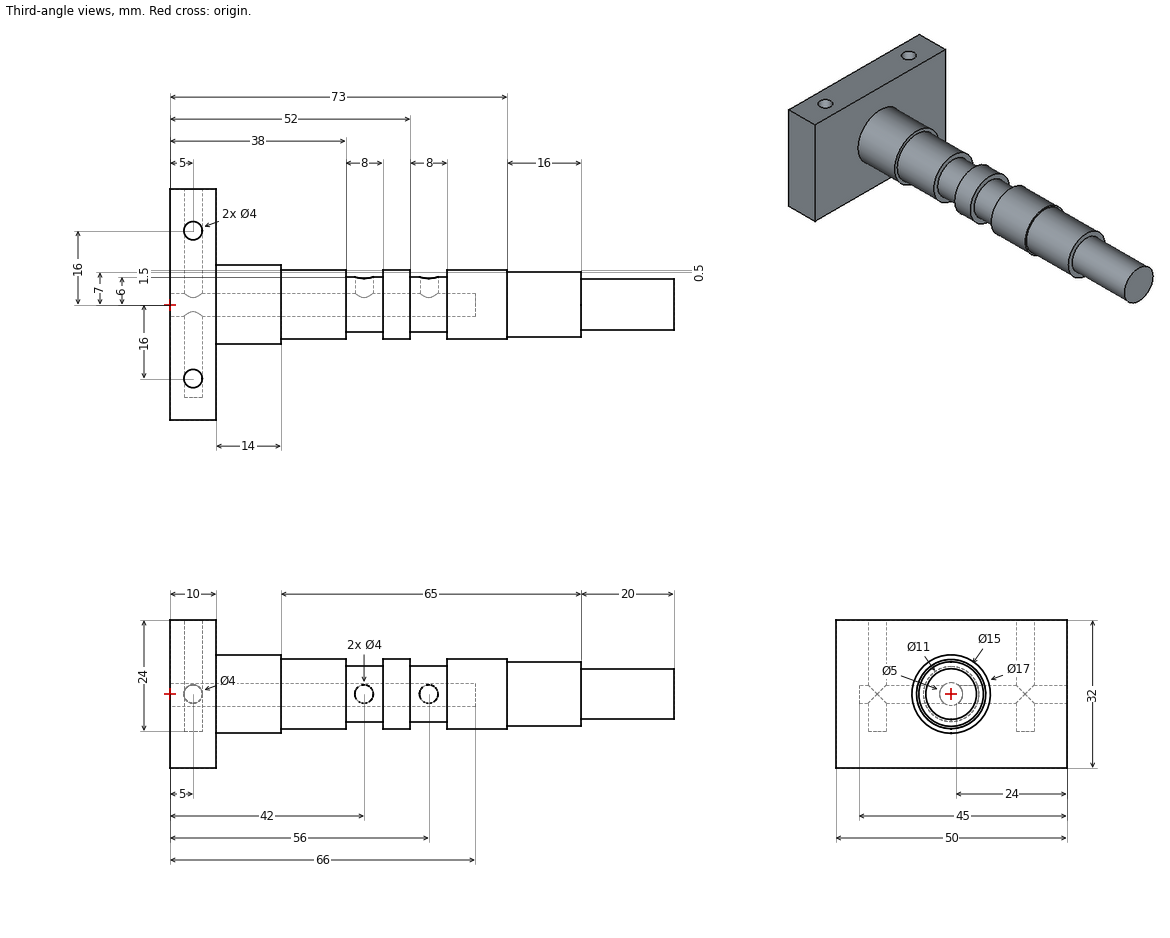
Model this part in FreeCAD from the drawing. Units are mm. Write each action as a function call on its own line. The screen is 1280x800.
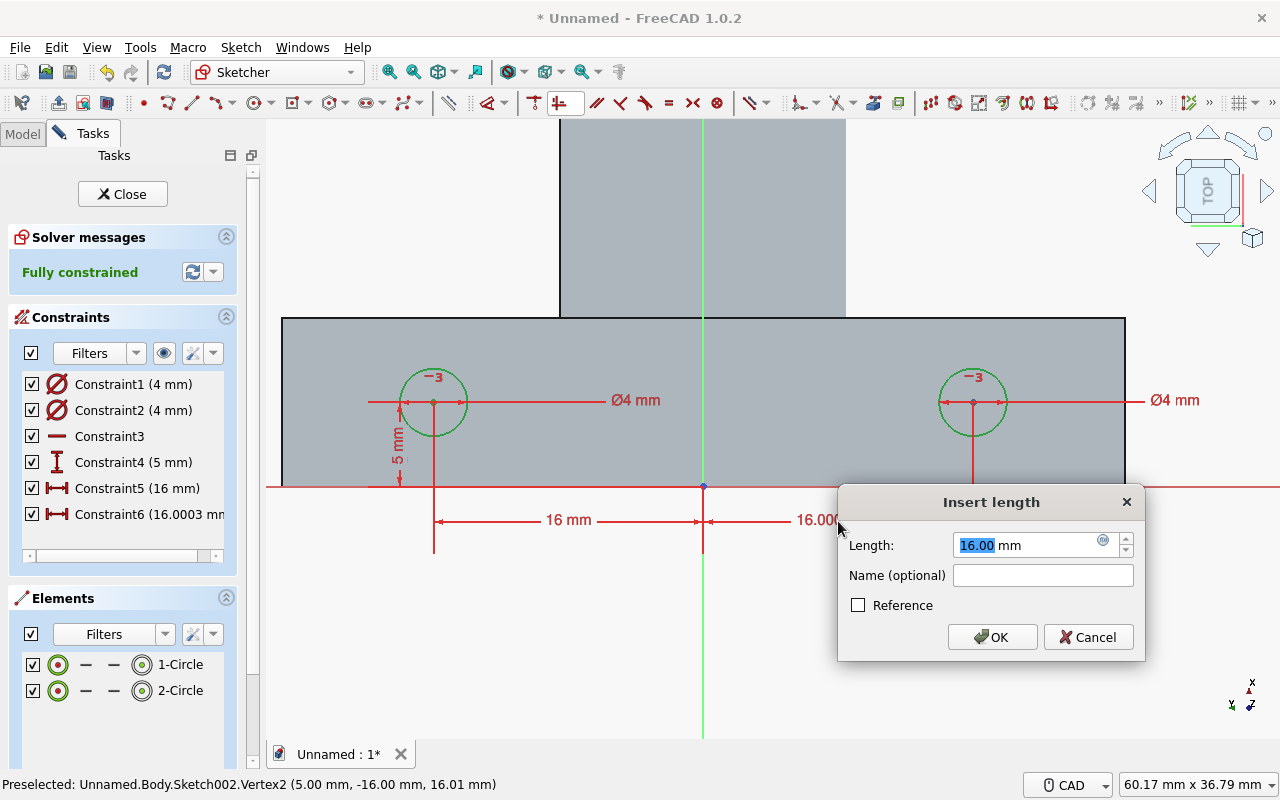
text(16)
key(Return)
key(Escape)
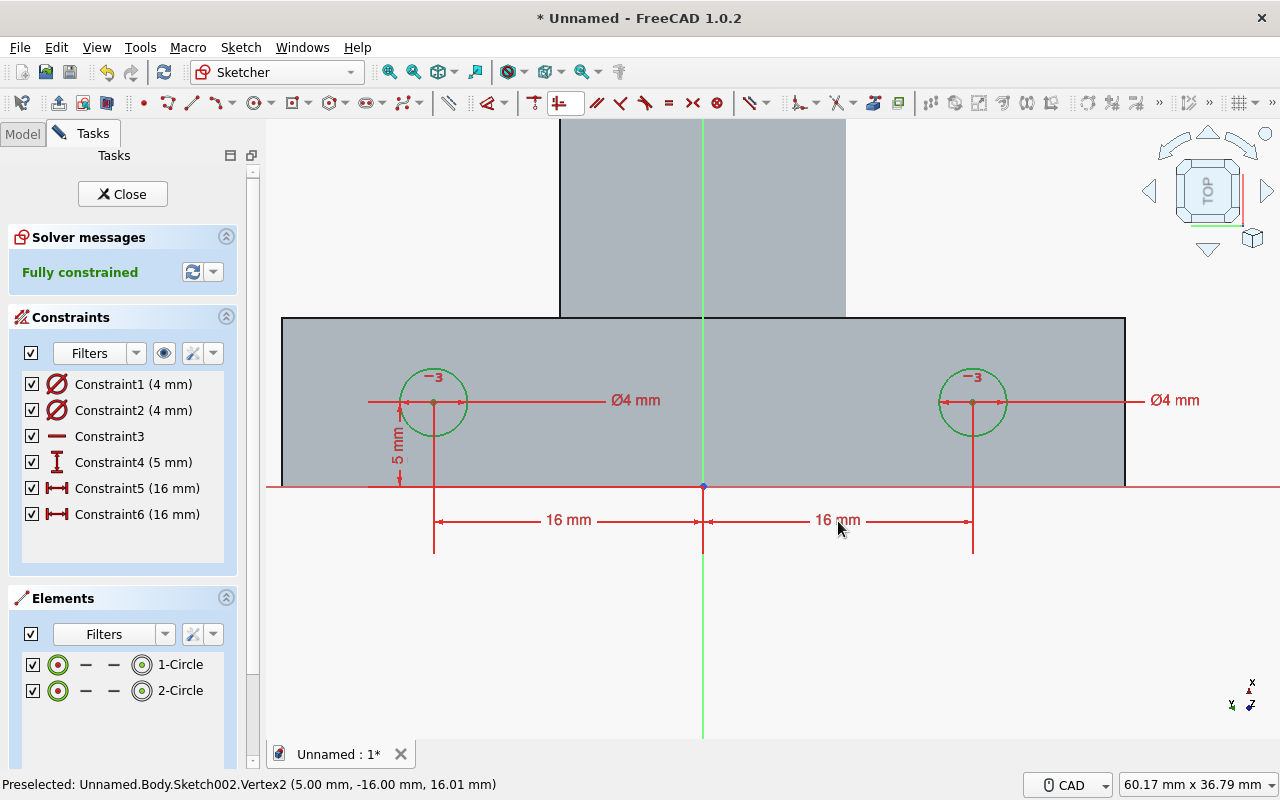
click(123, 194)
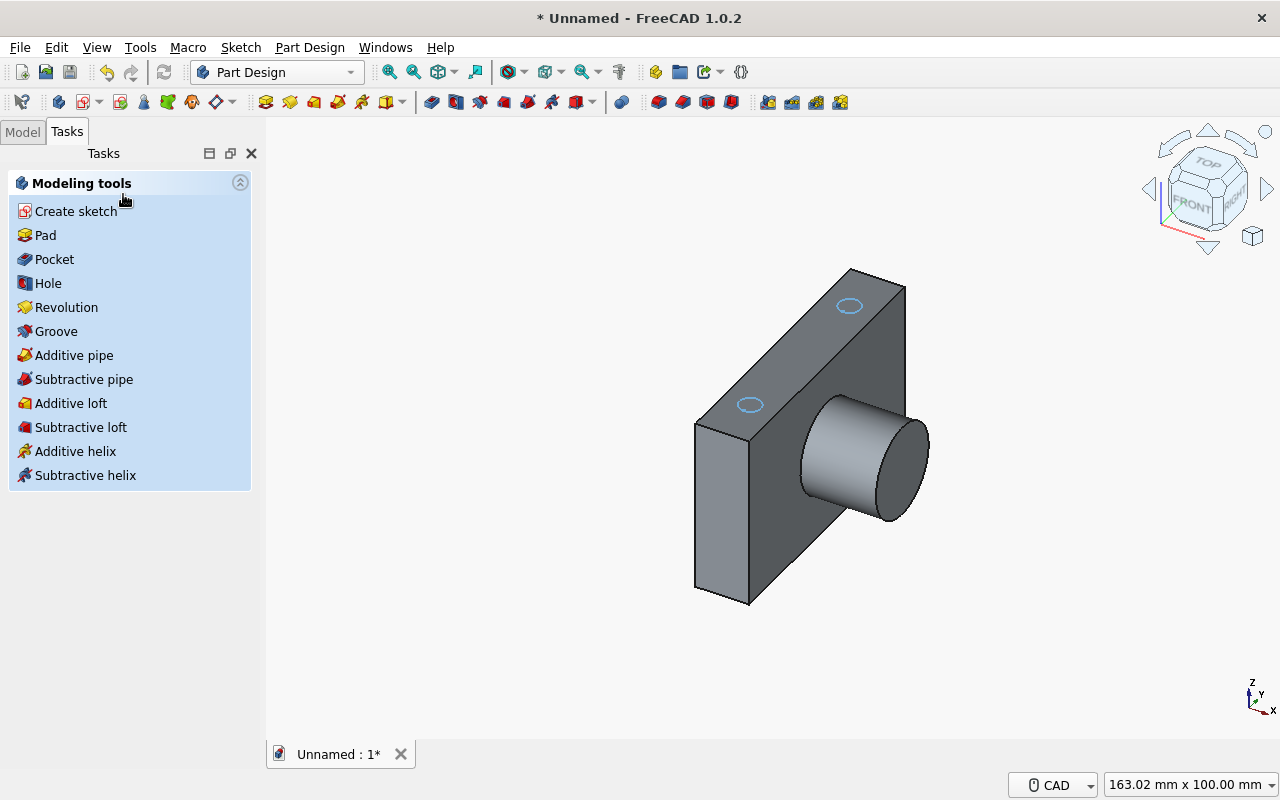
click(432, 102)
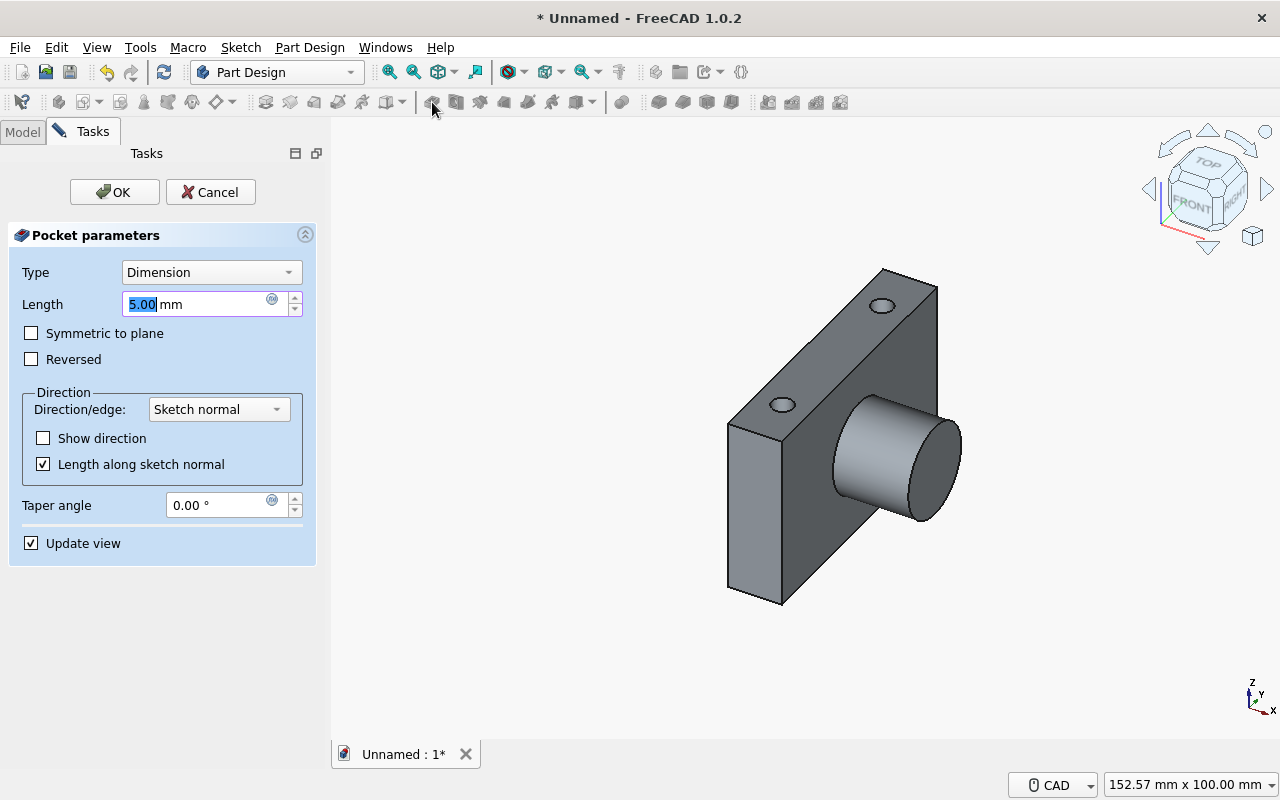
text(24)
key(Tab)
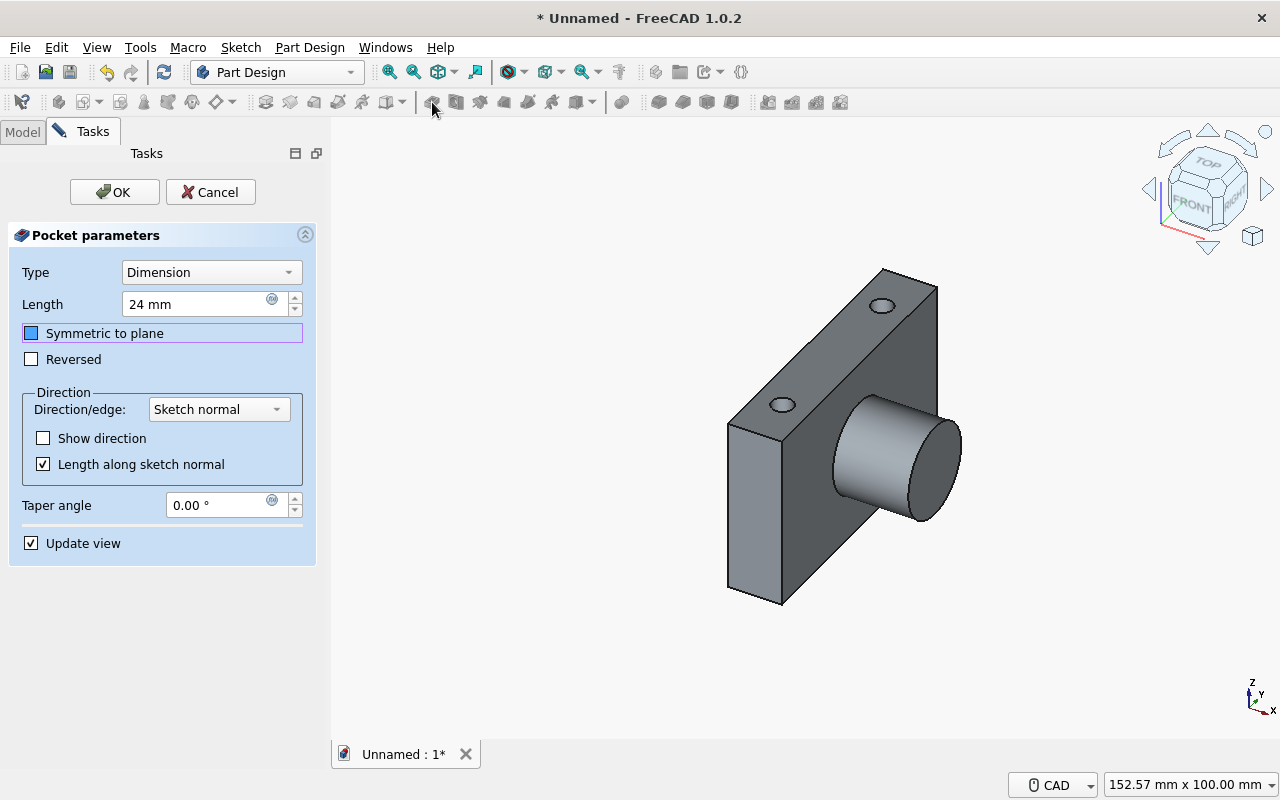
click(115, 192)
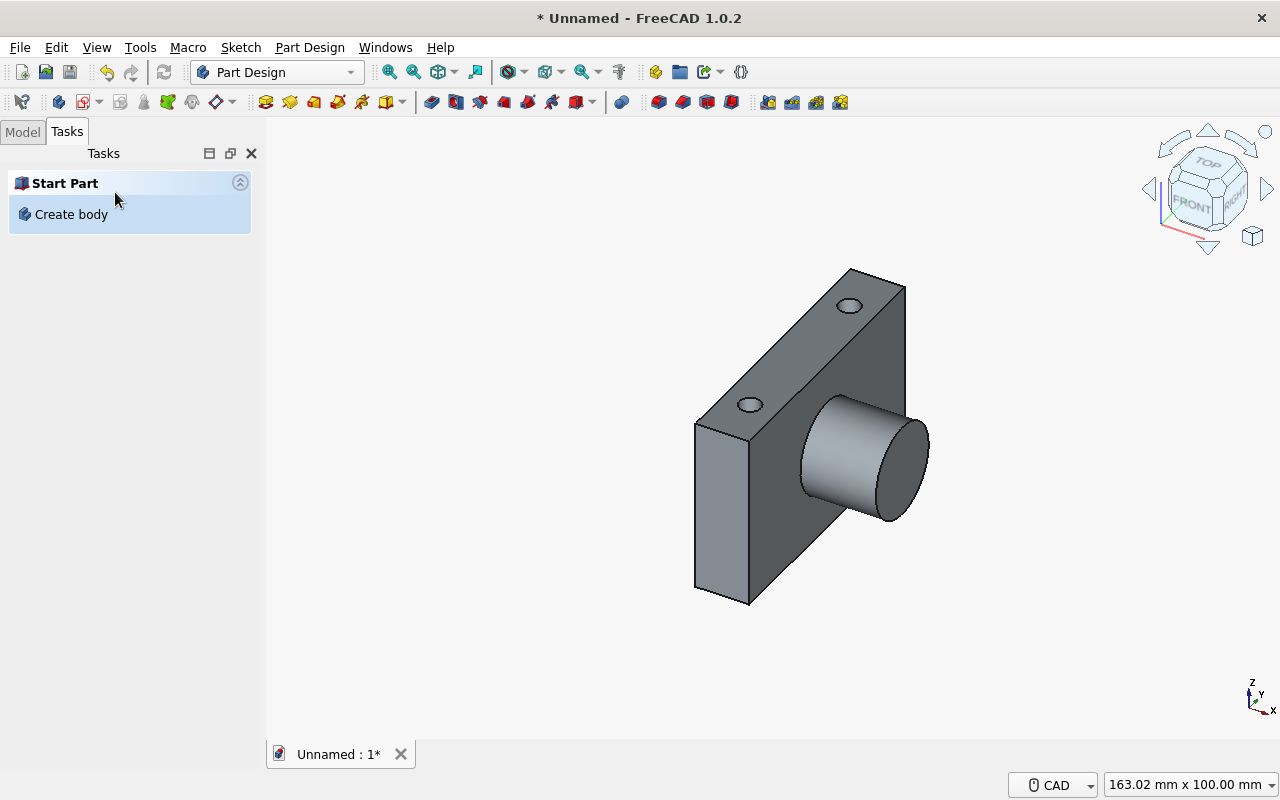
key(4)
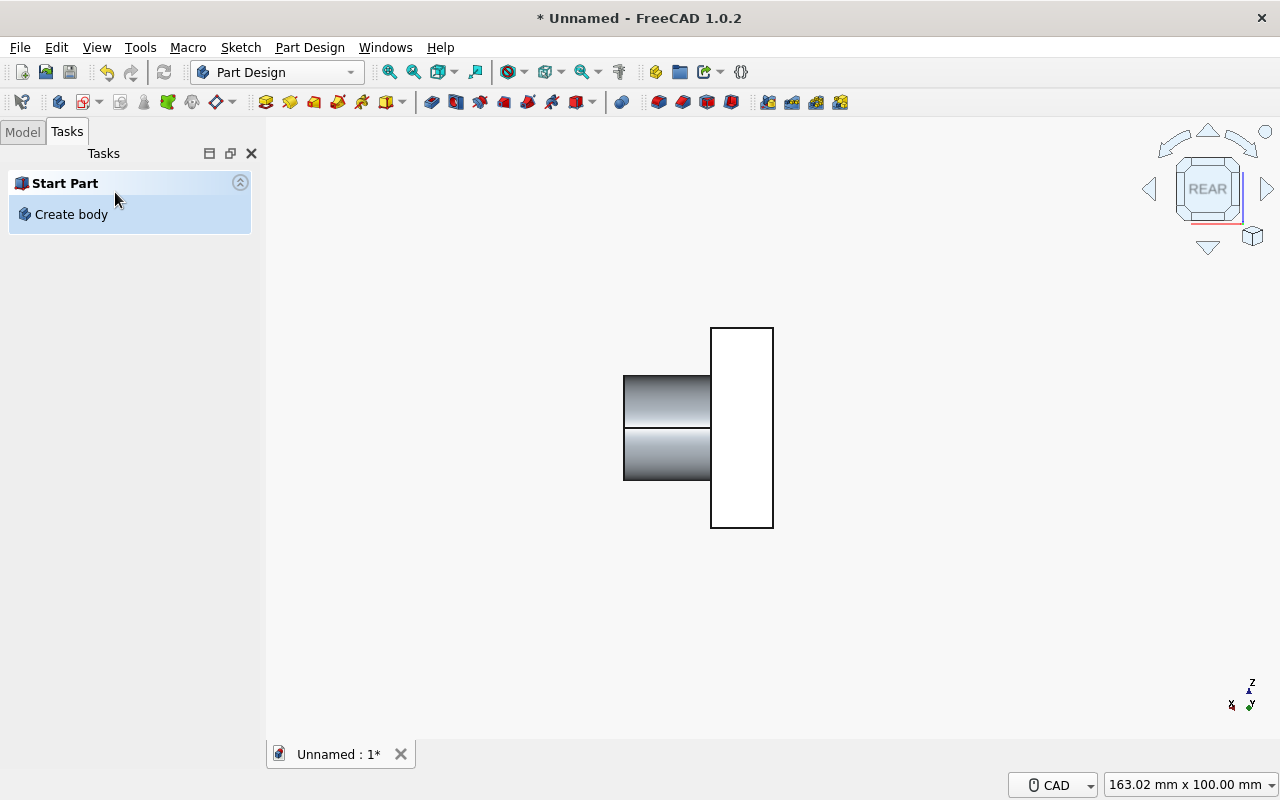
click(390, 72)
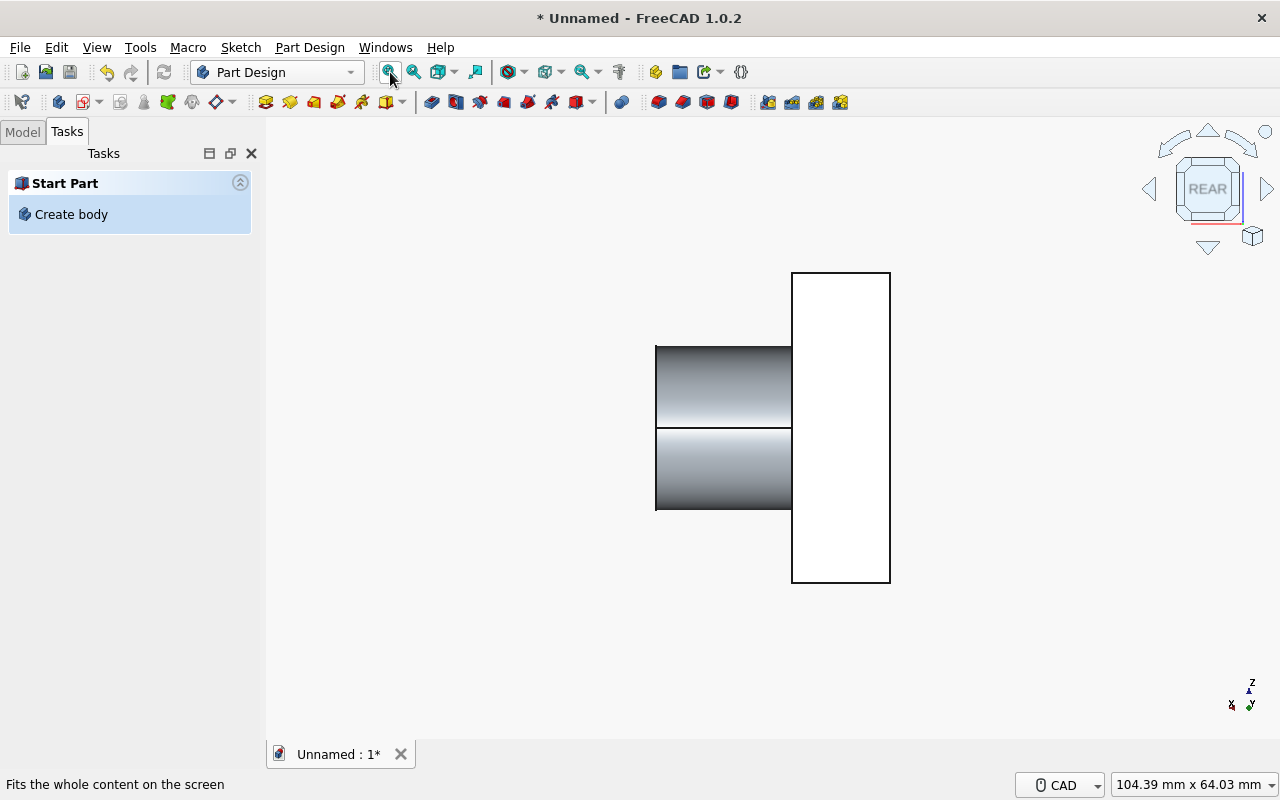
click(841, 471)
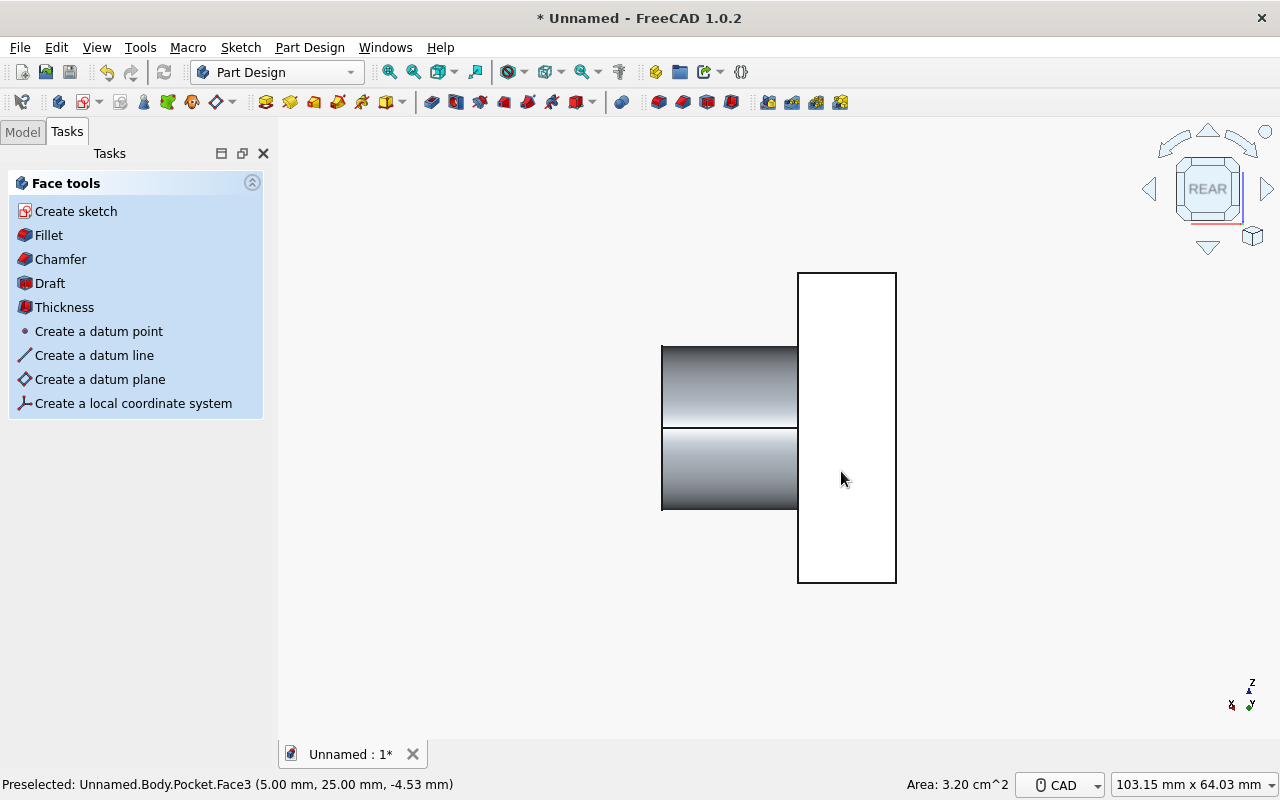
click(84, 102)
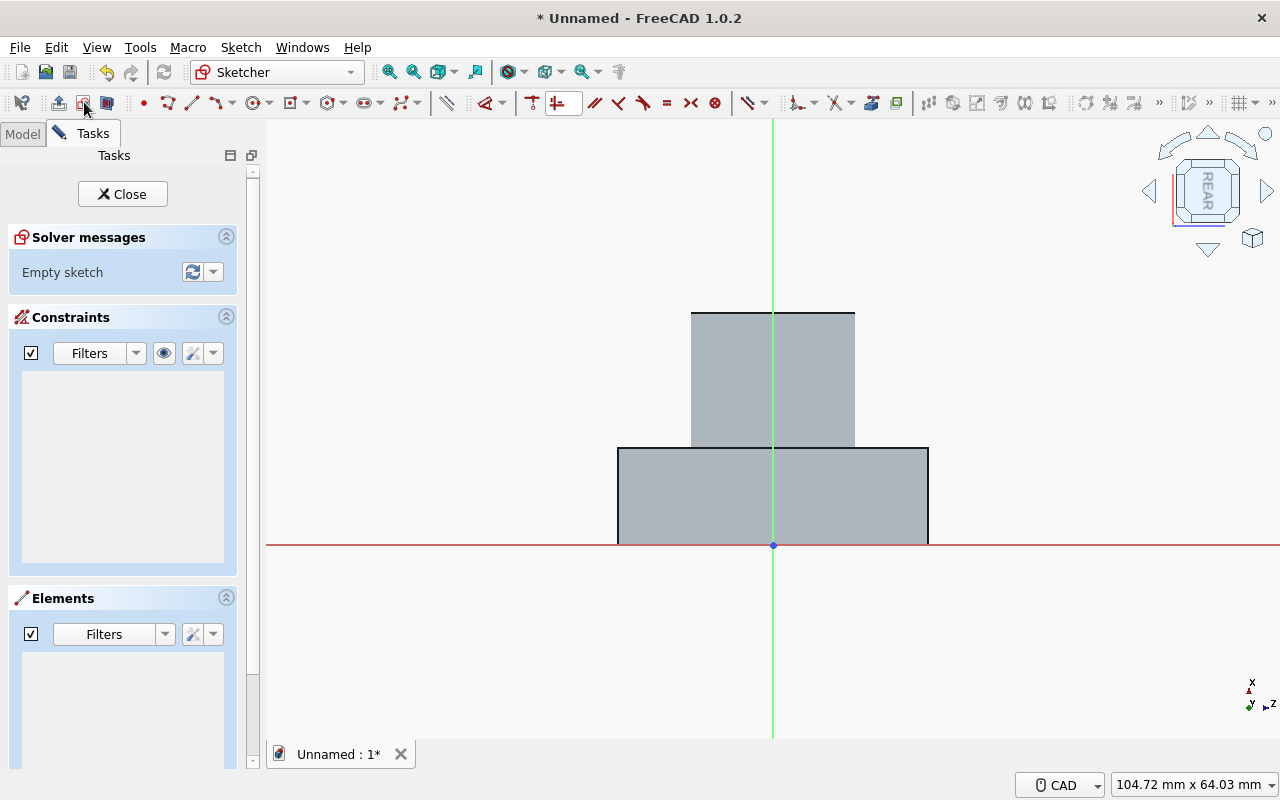
scroll(787, 528, up, 9)